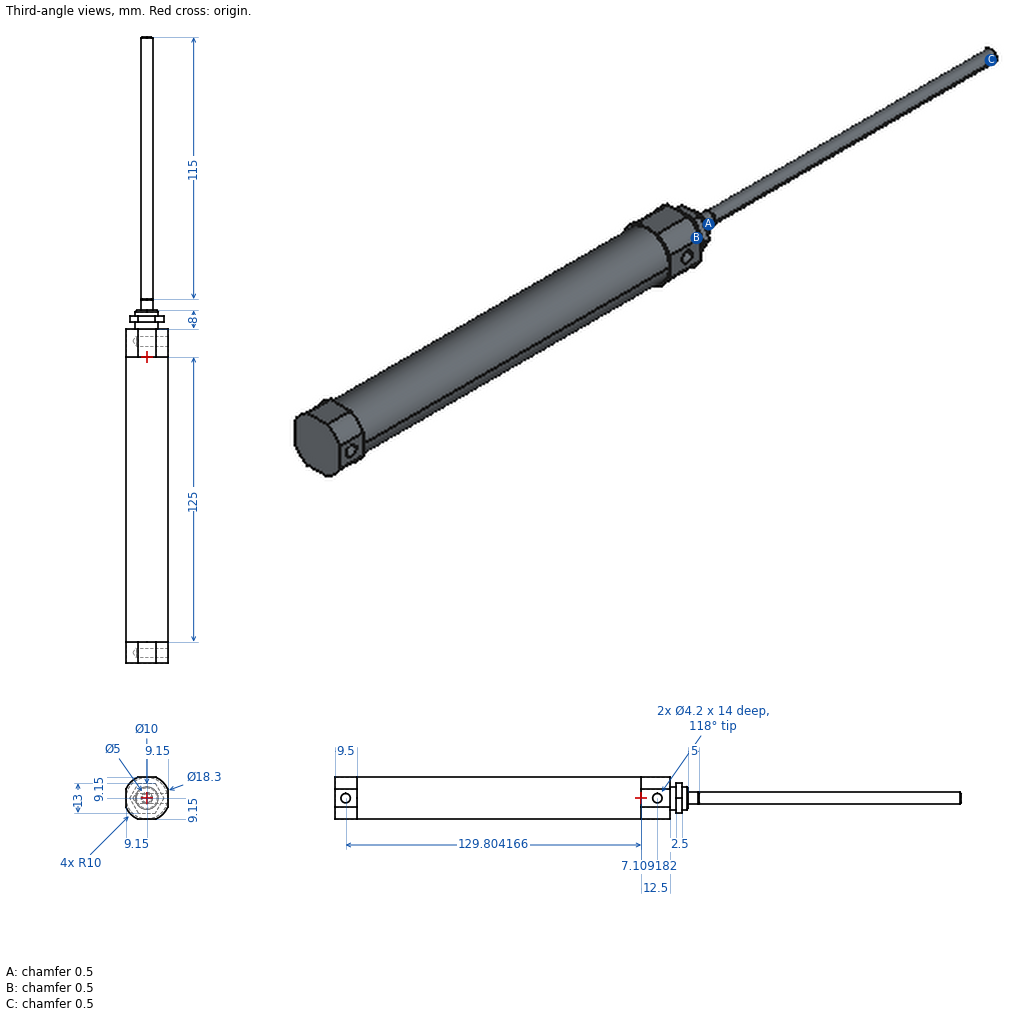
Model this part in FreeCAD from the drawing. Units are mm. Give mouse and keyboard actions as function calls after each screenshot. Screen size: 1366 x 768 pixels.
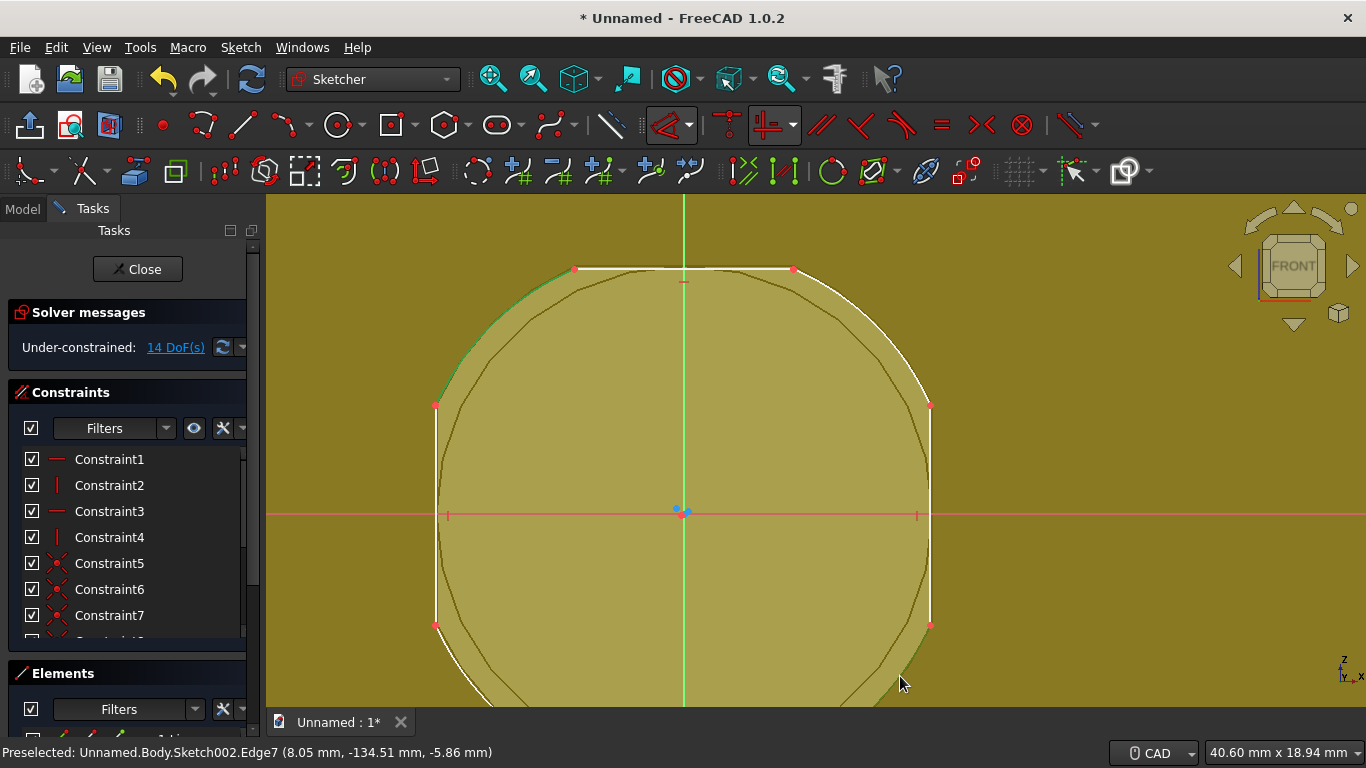
key(c)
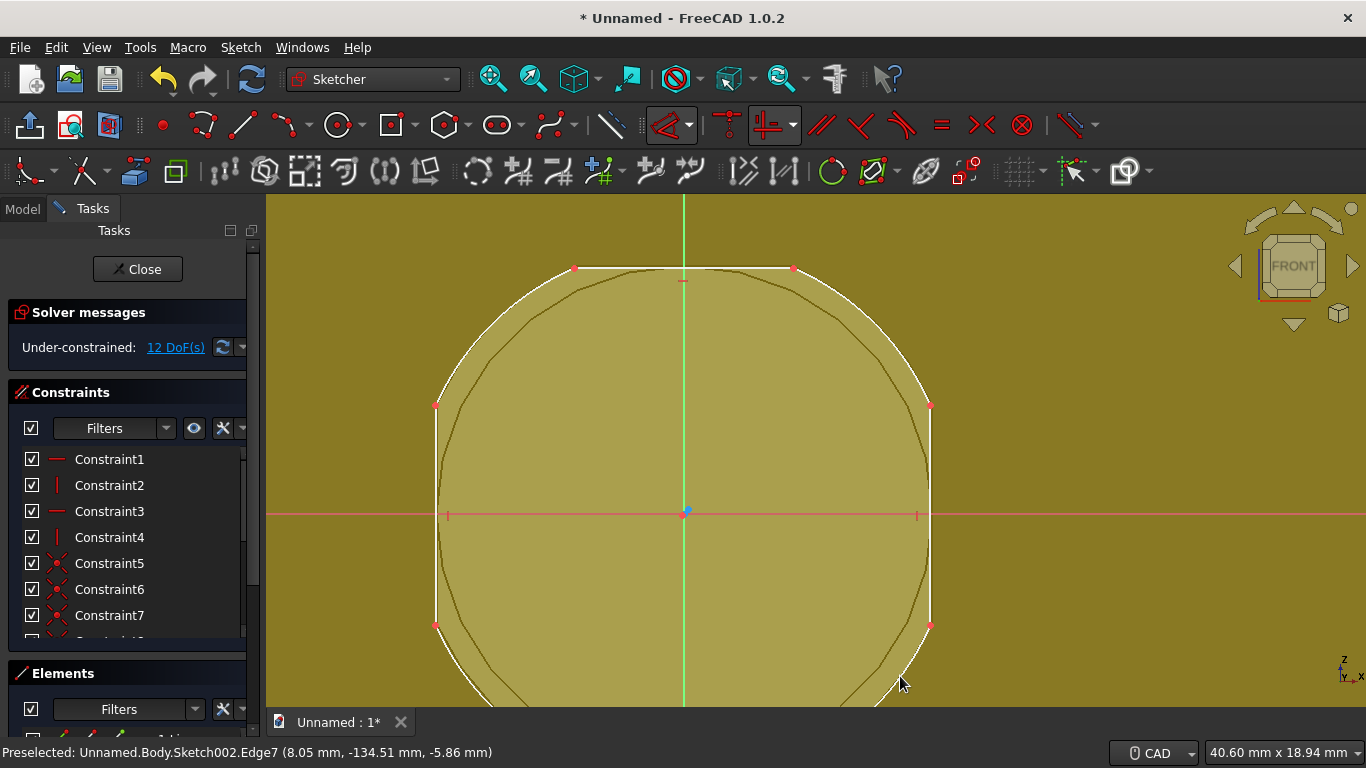
click(522, 298)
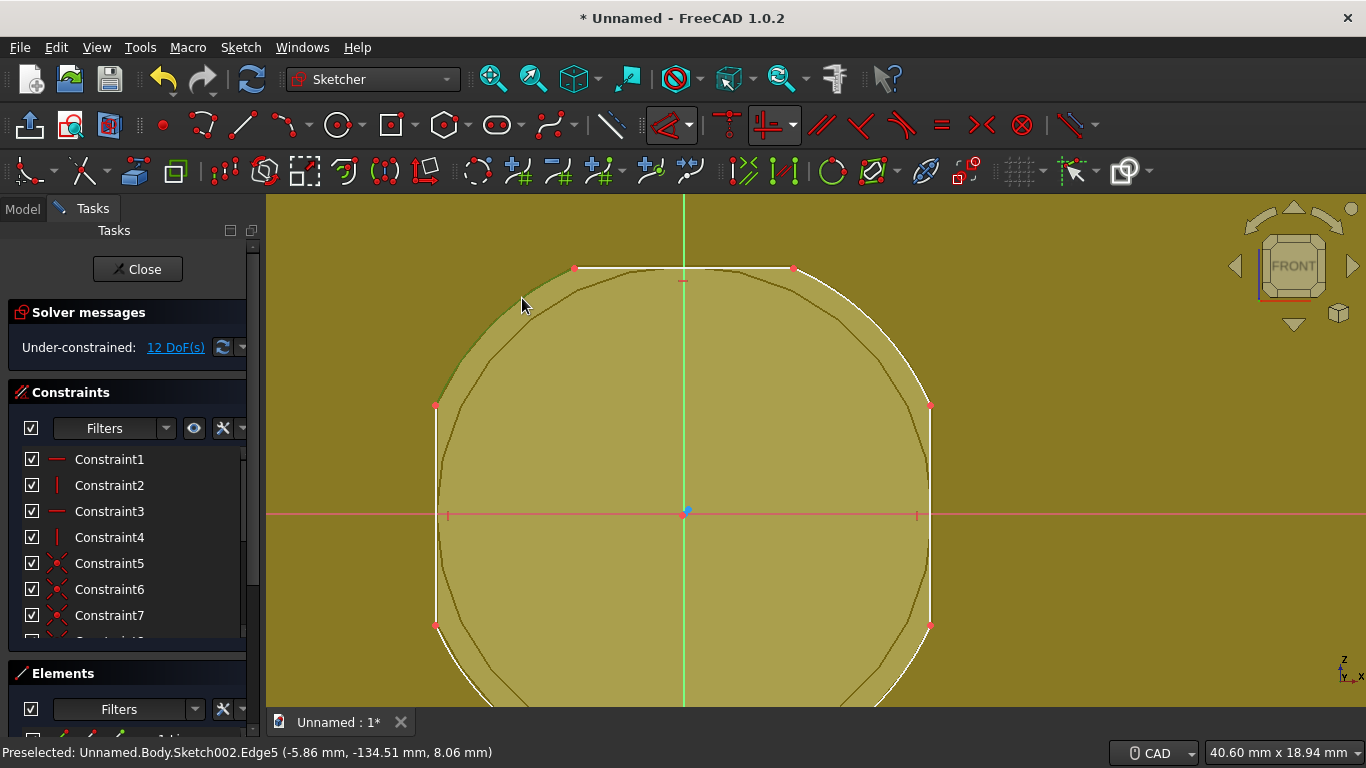
click(901, 354)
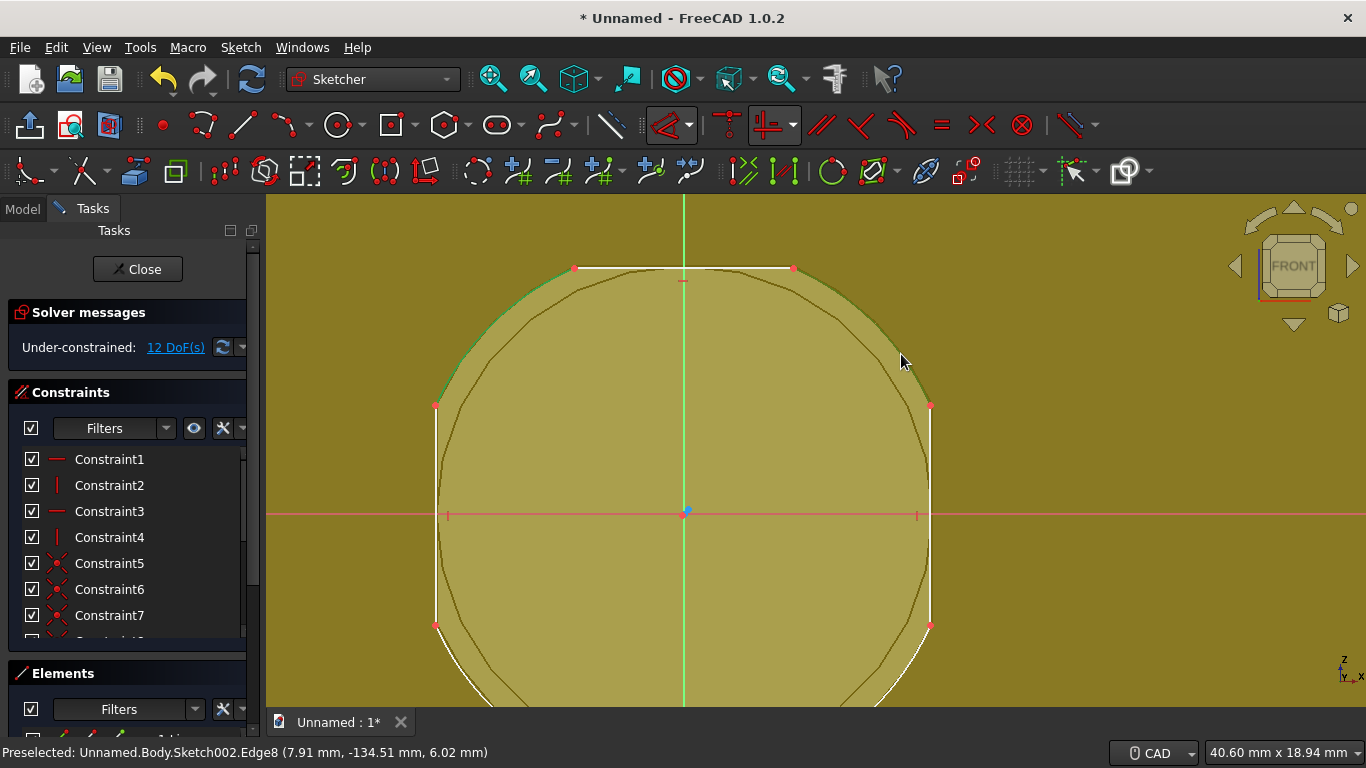
key(c)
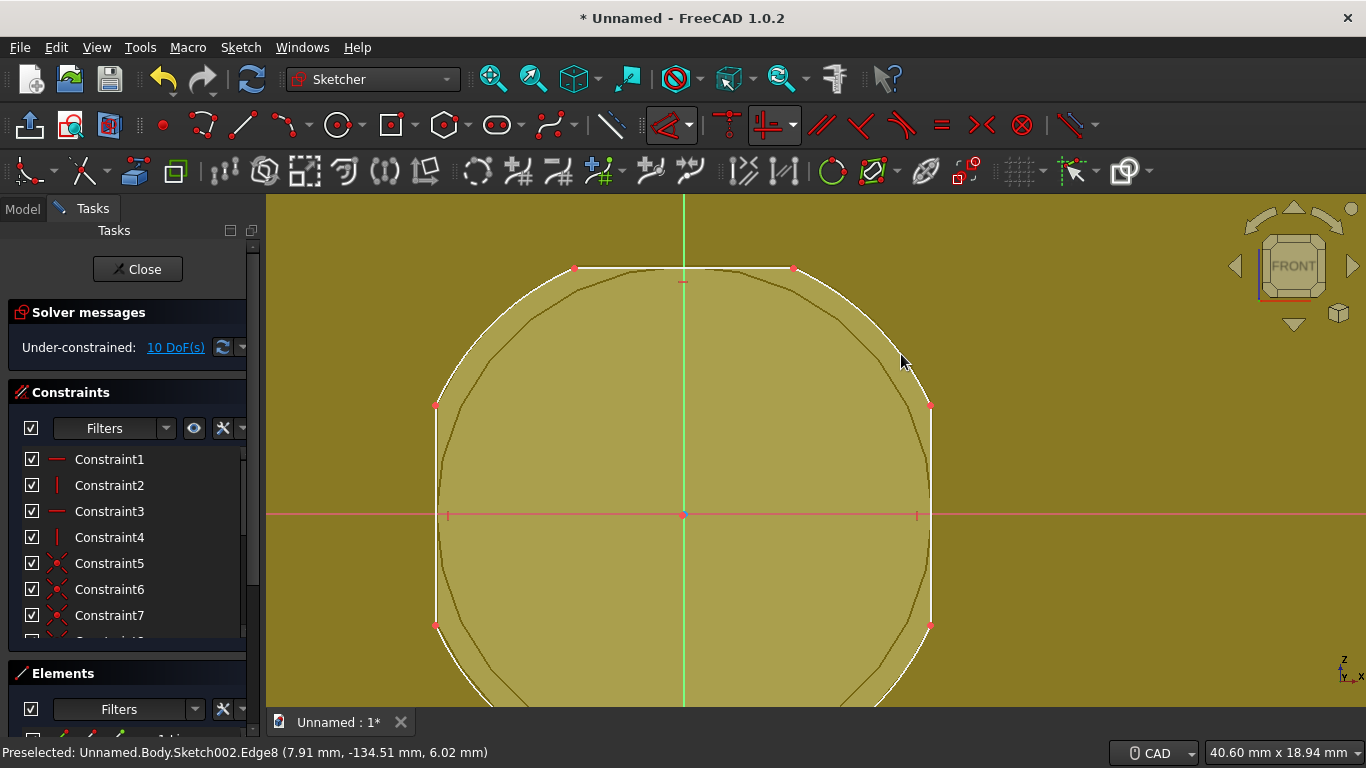
drag(673, 504, 694, 525)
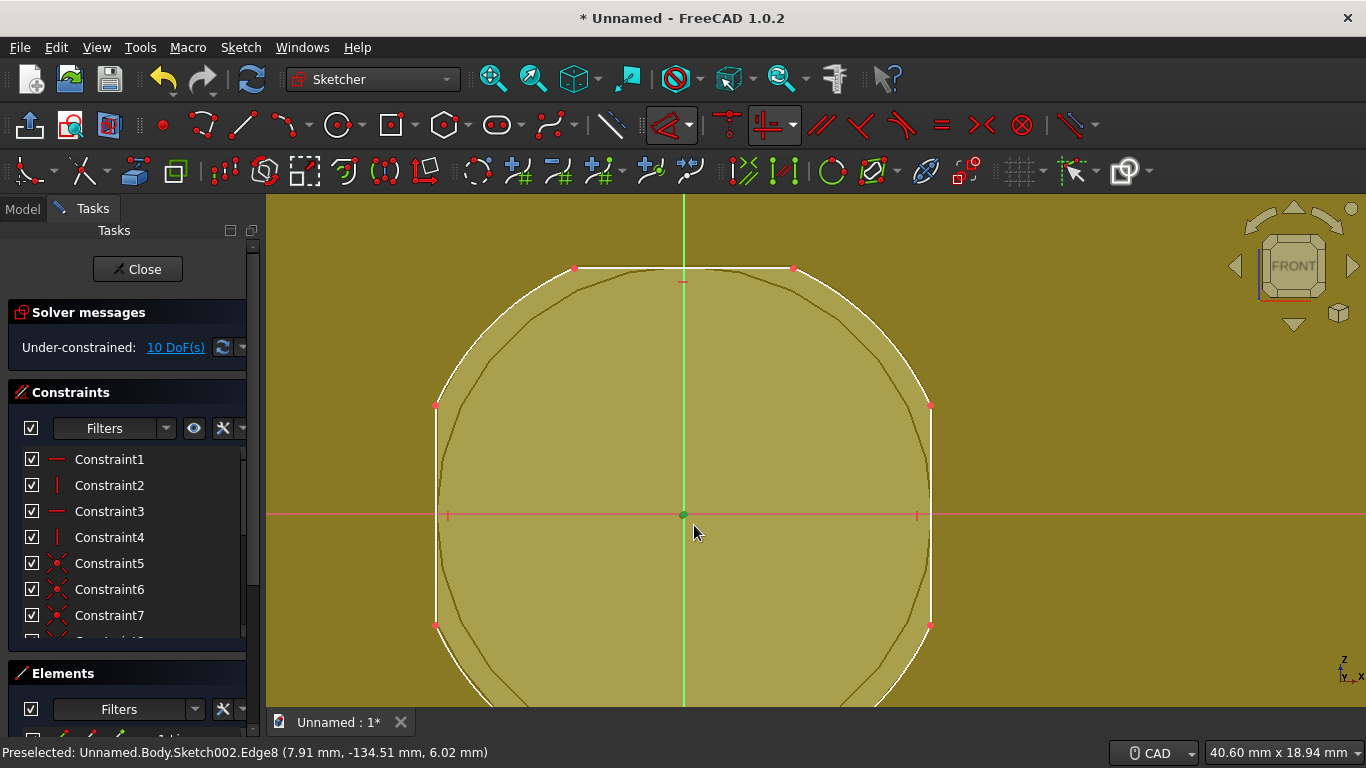
key(c)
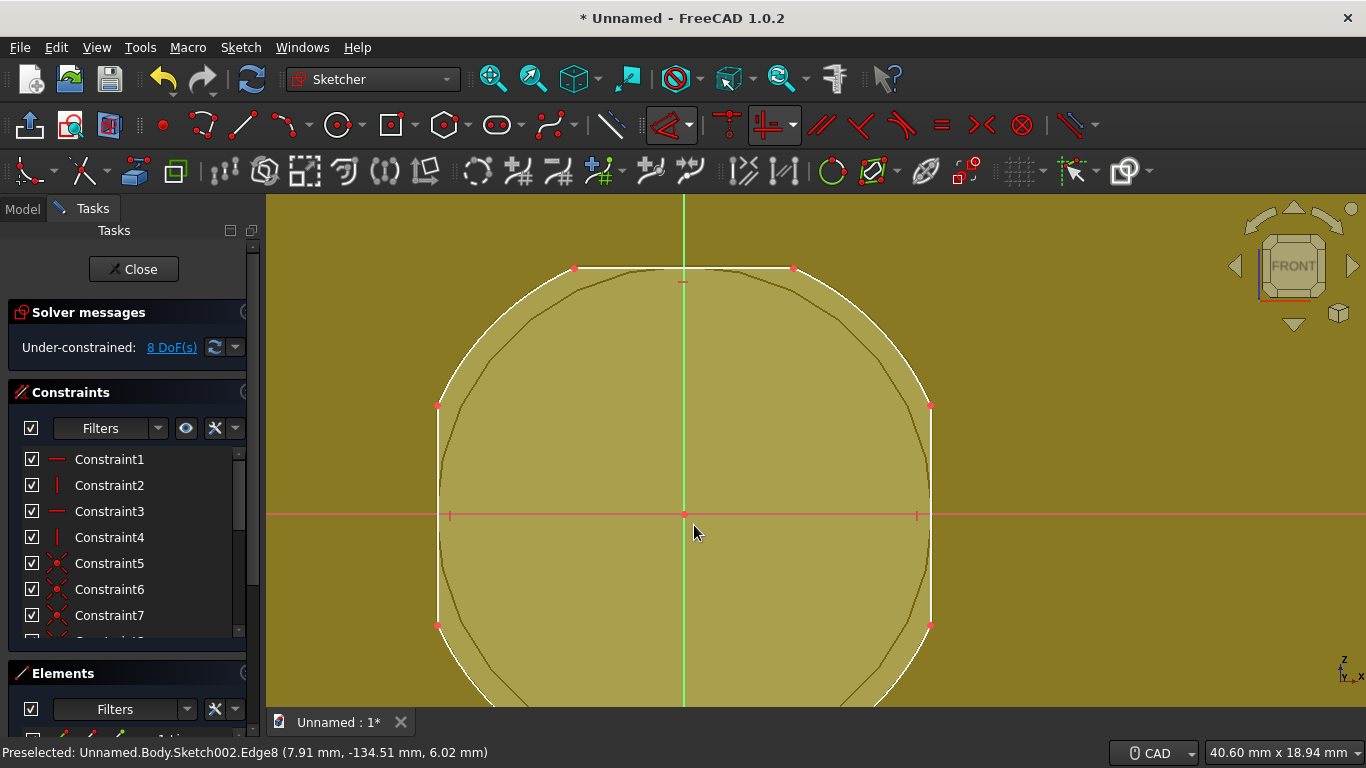
click(523, 298)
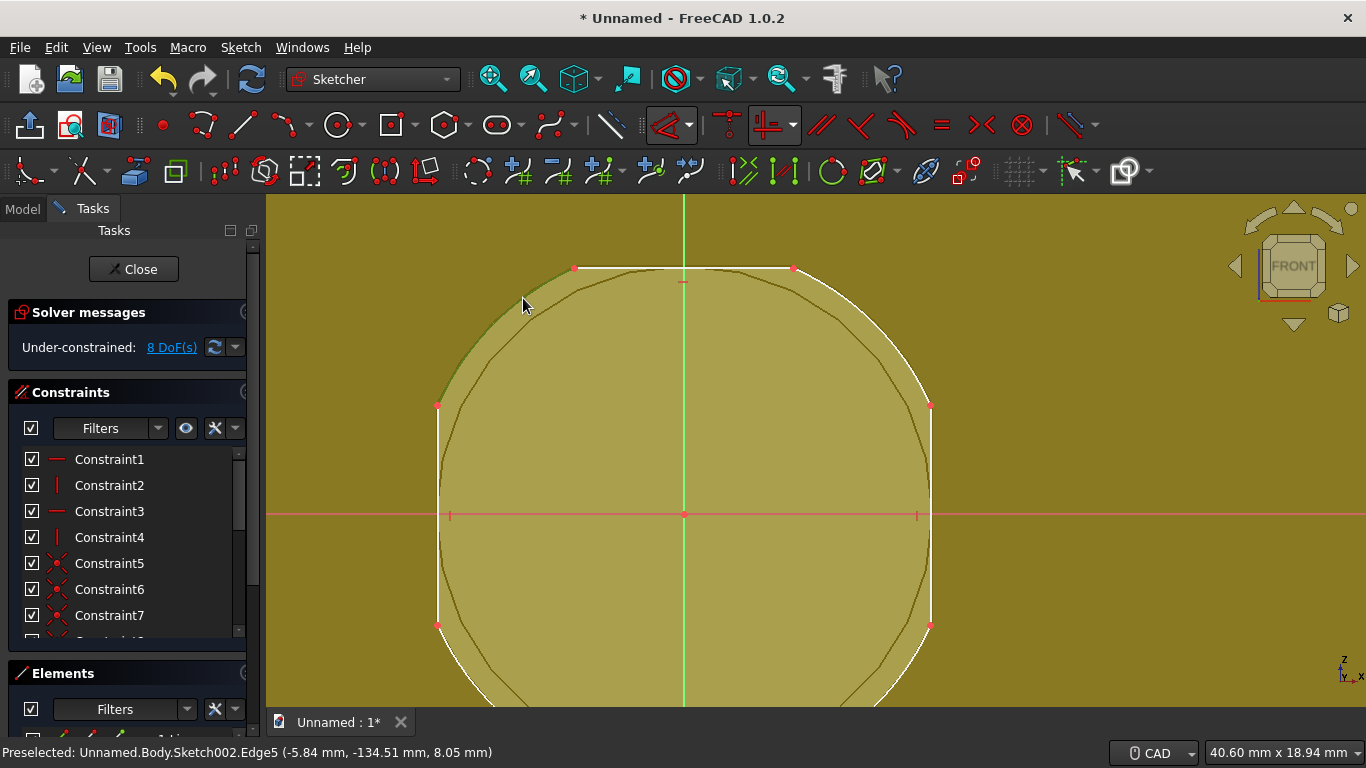
click(468, 676)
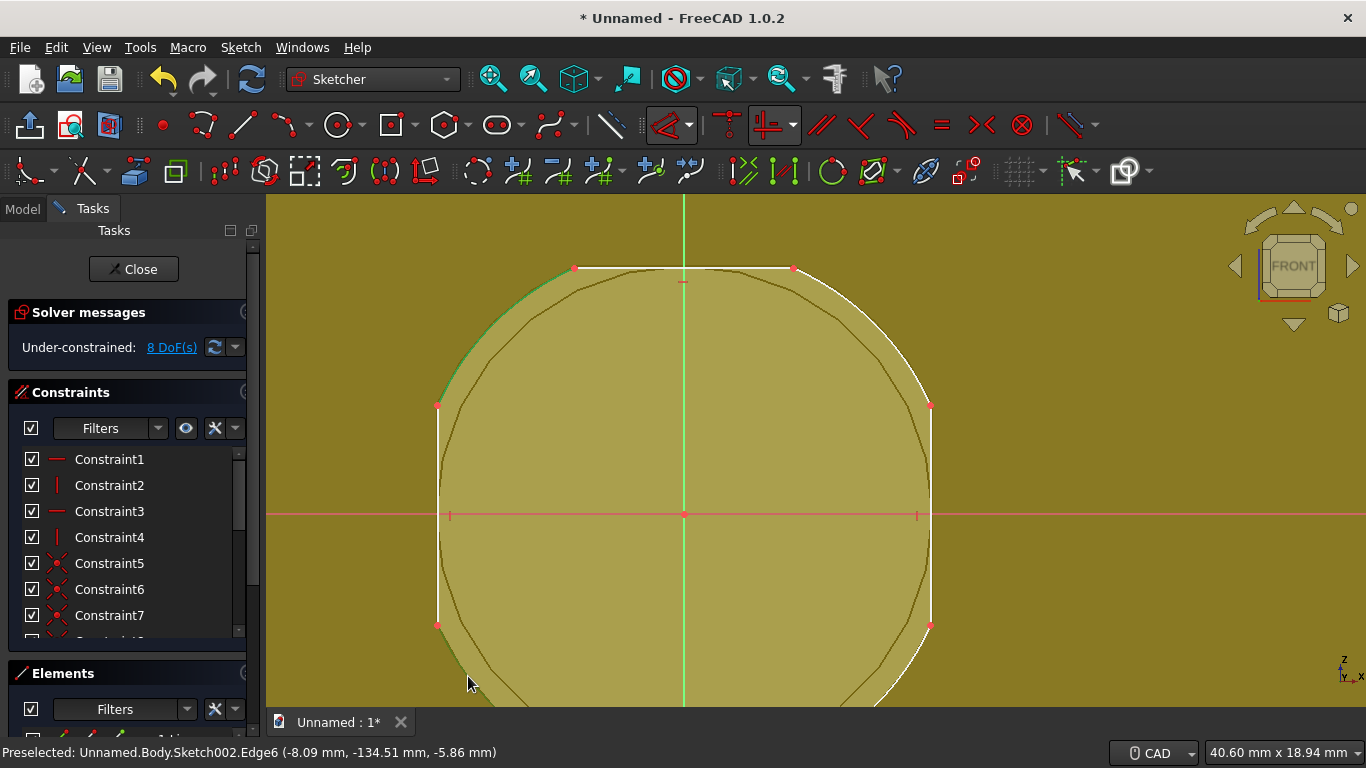
click(901, 676)